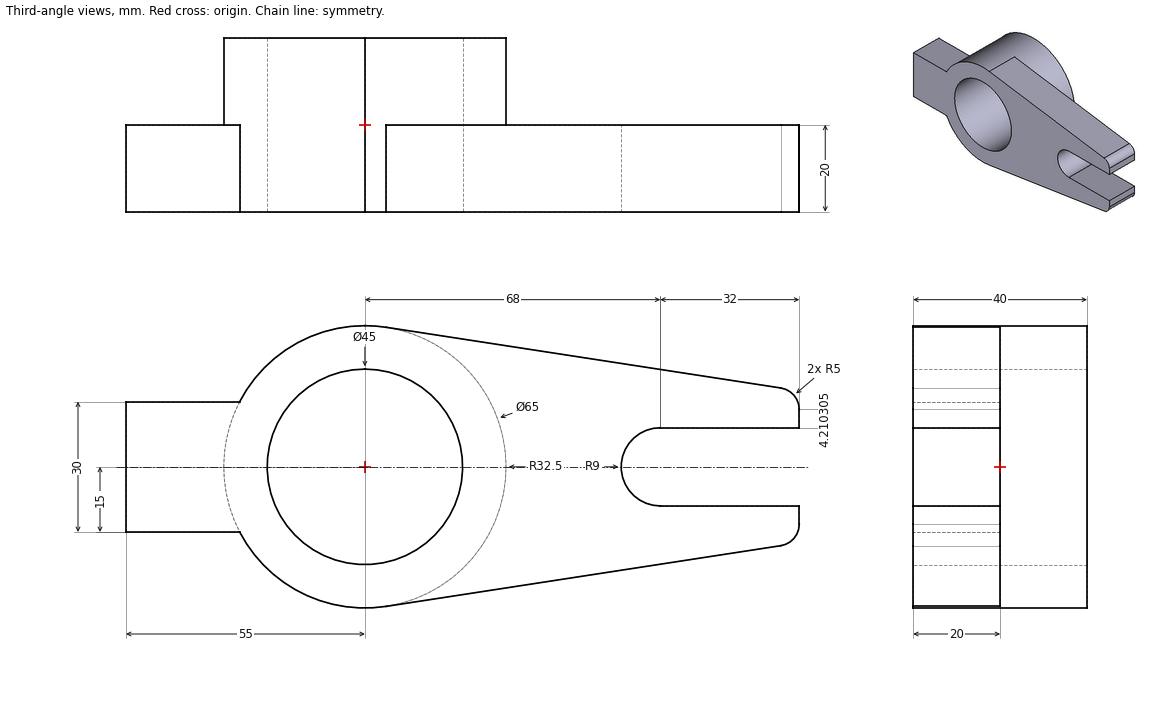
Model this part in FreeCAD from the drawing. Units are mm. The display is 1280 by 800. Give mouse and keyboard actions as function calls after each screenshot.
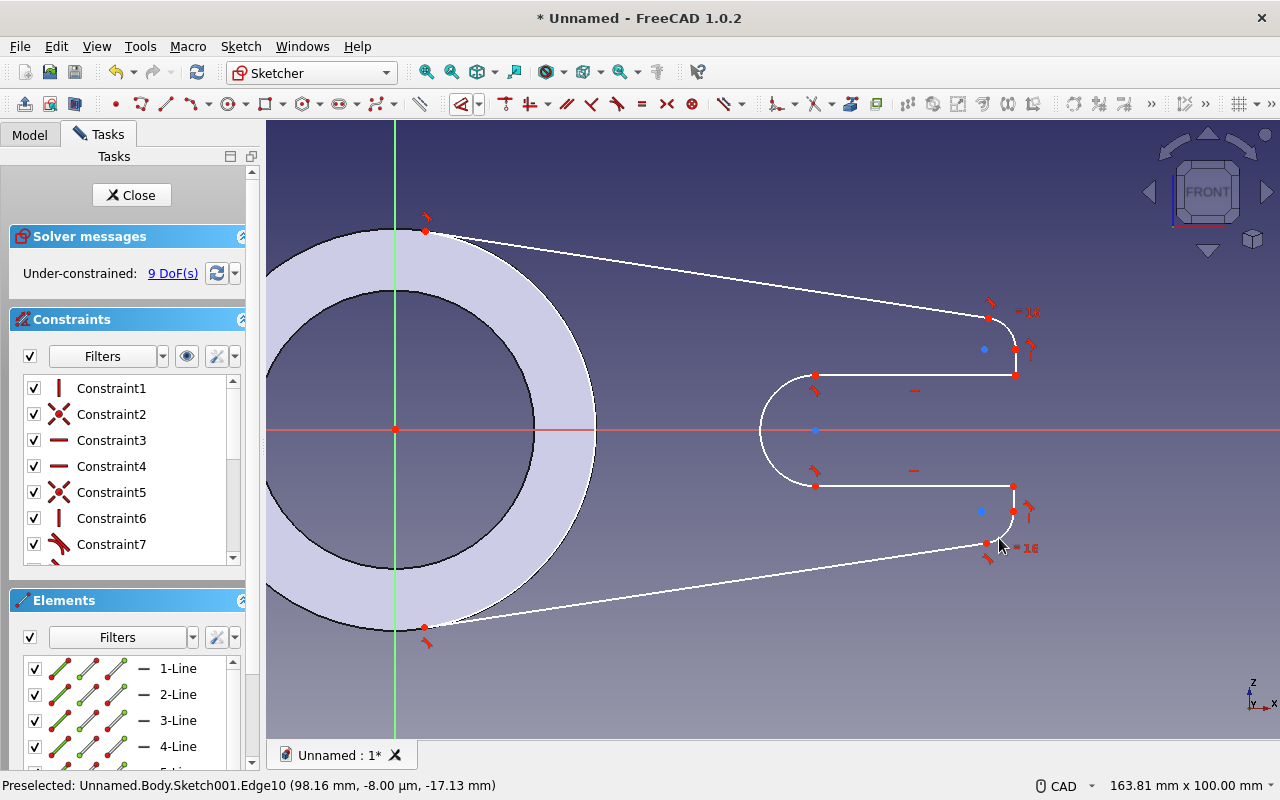
click(816, 431)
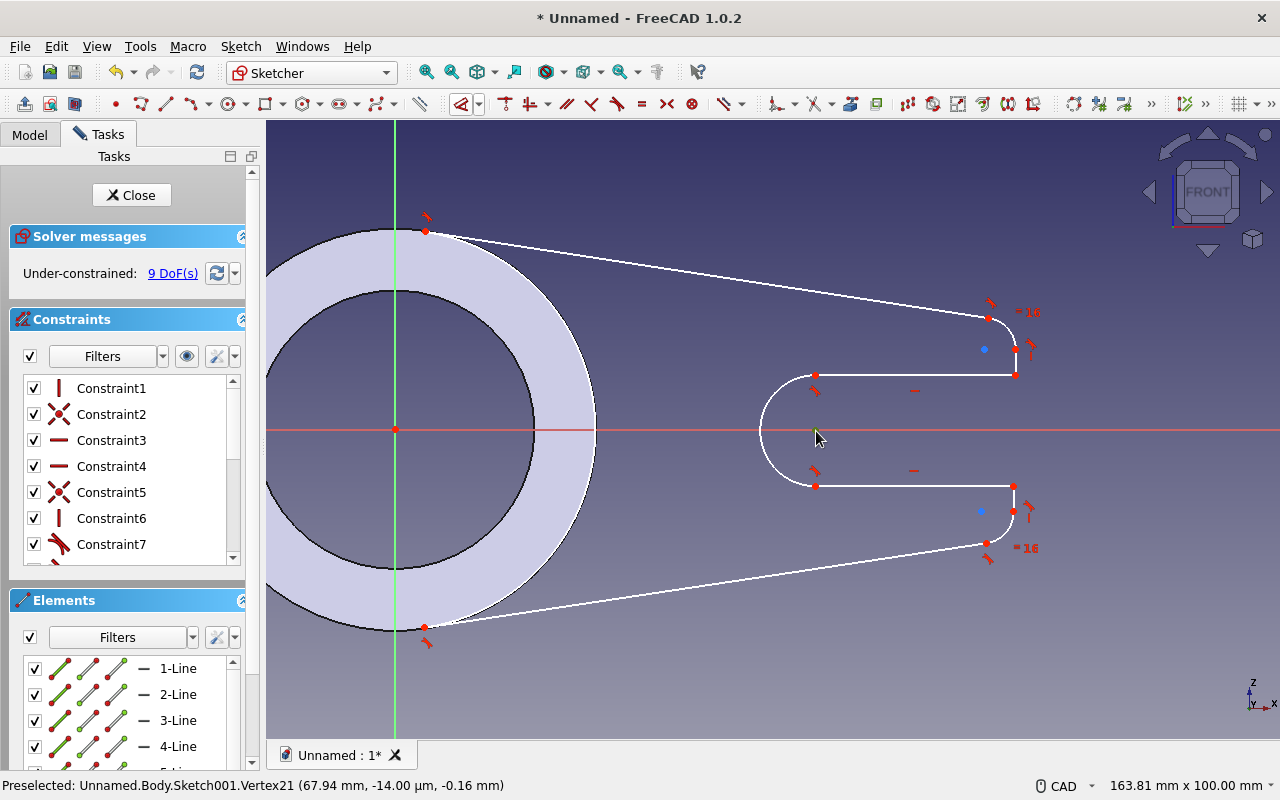
click(353, 430)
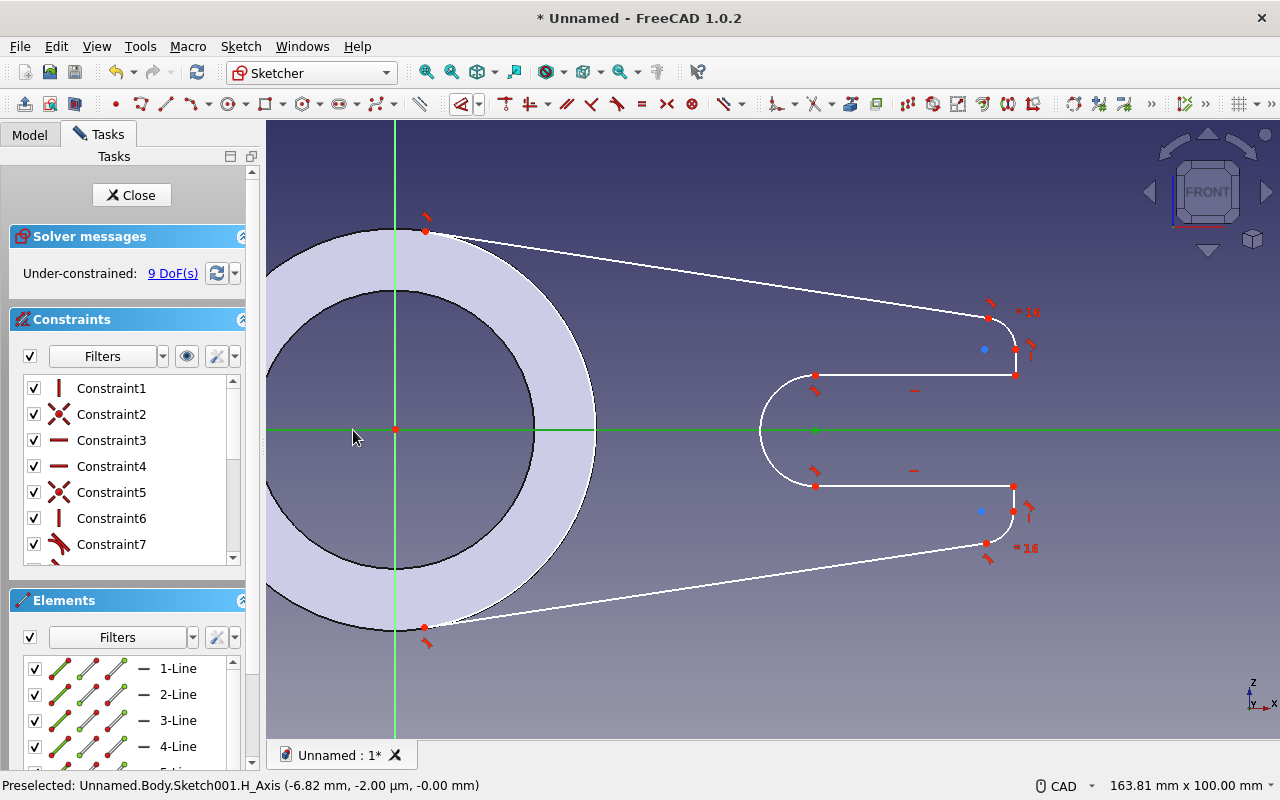
key(c)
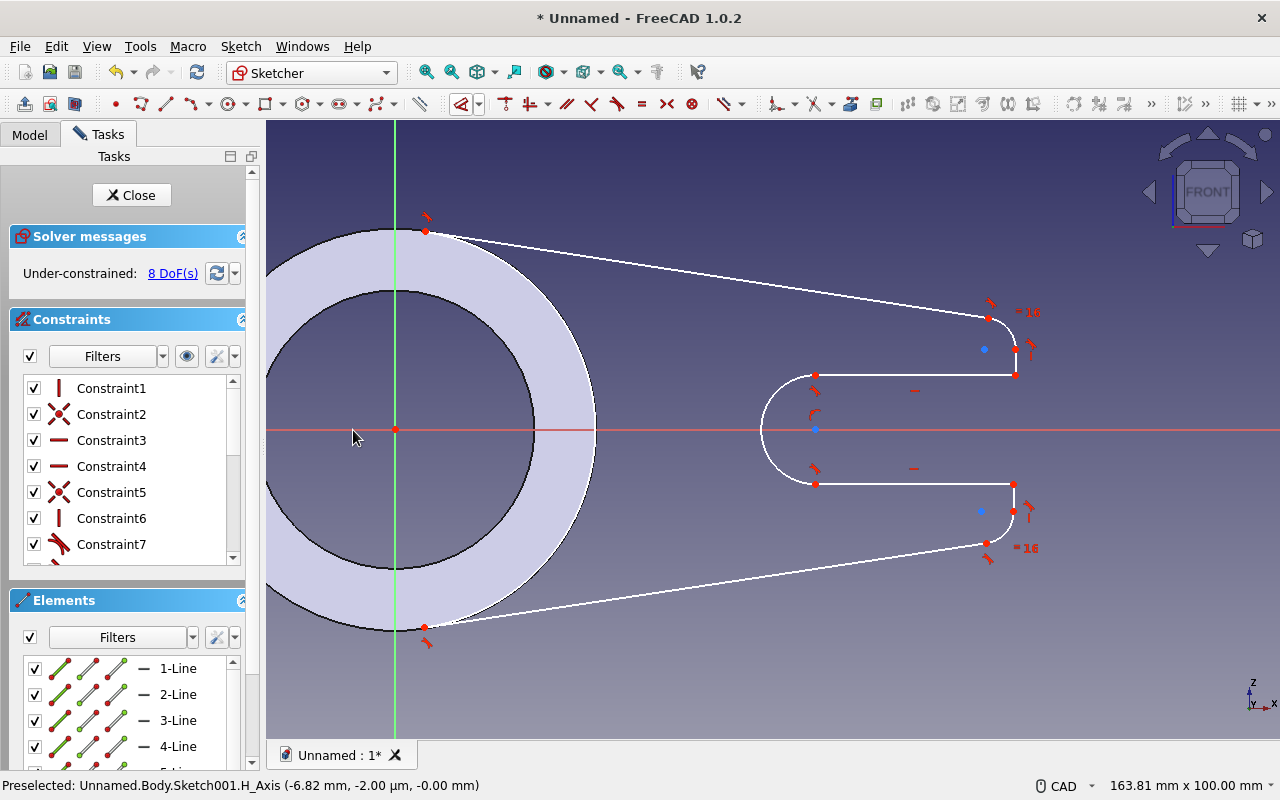
click(984, 349)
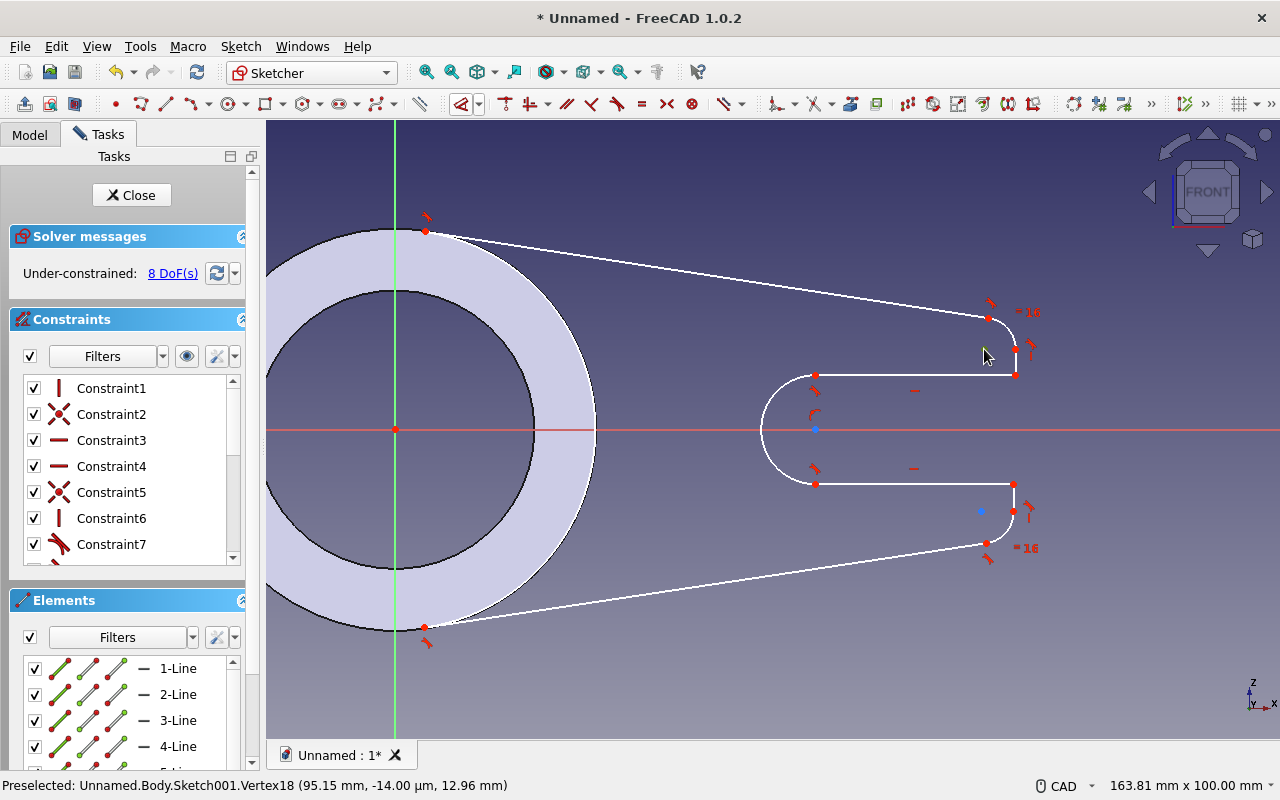
click(982, 512)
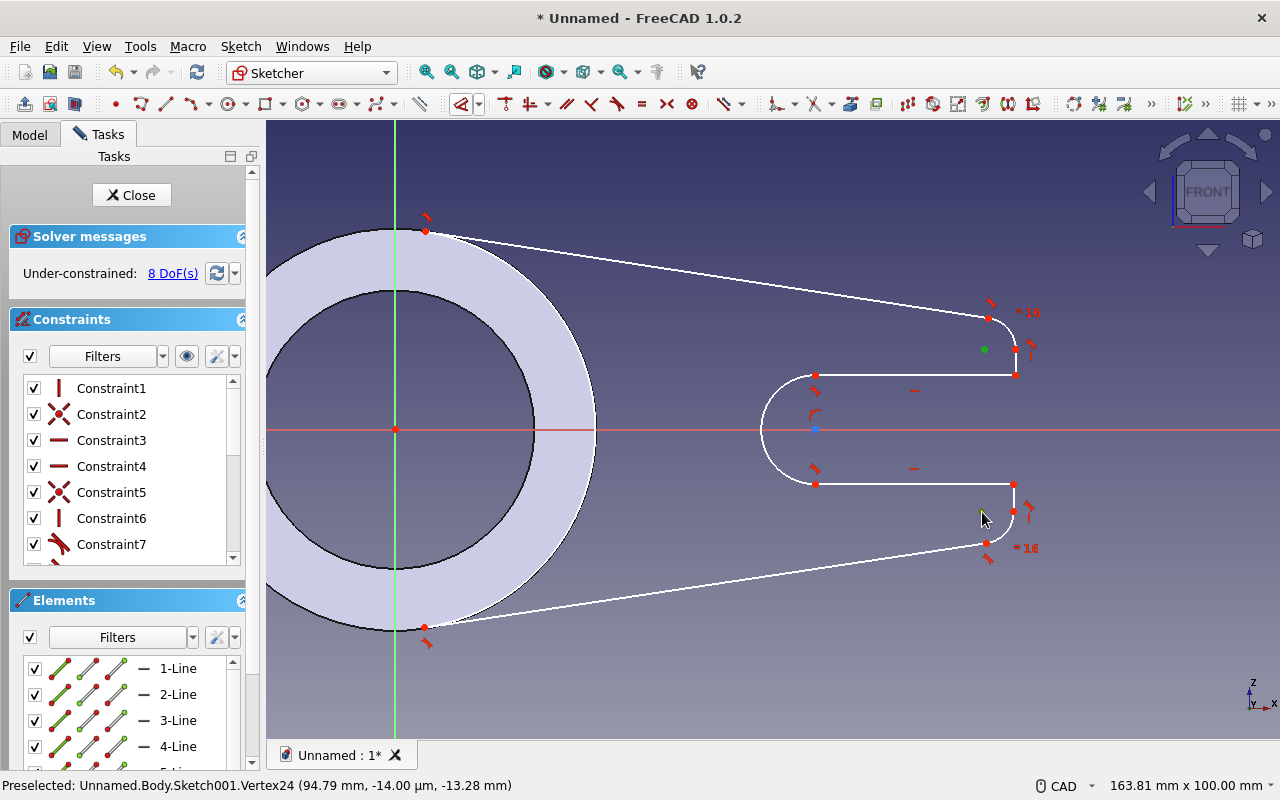
click(353, 430)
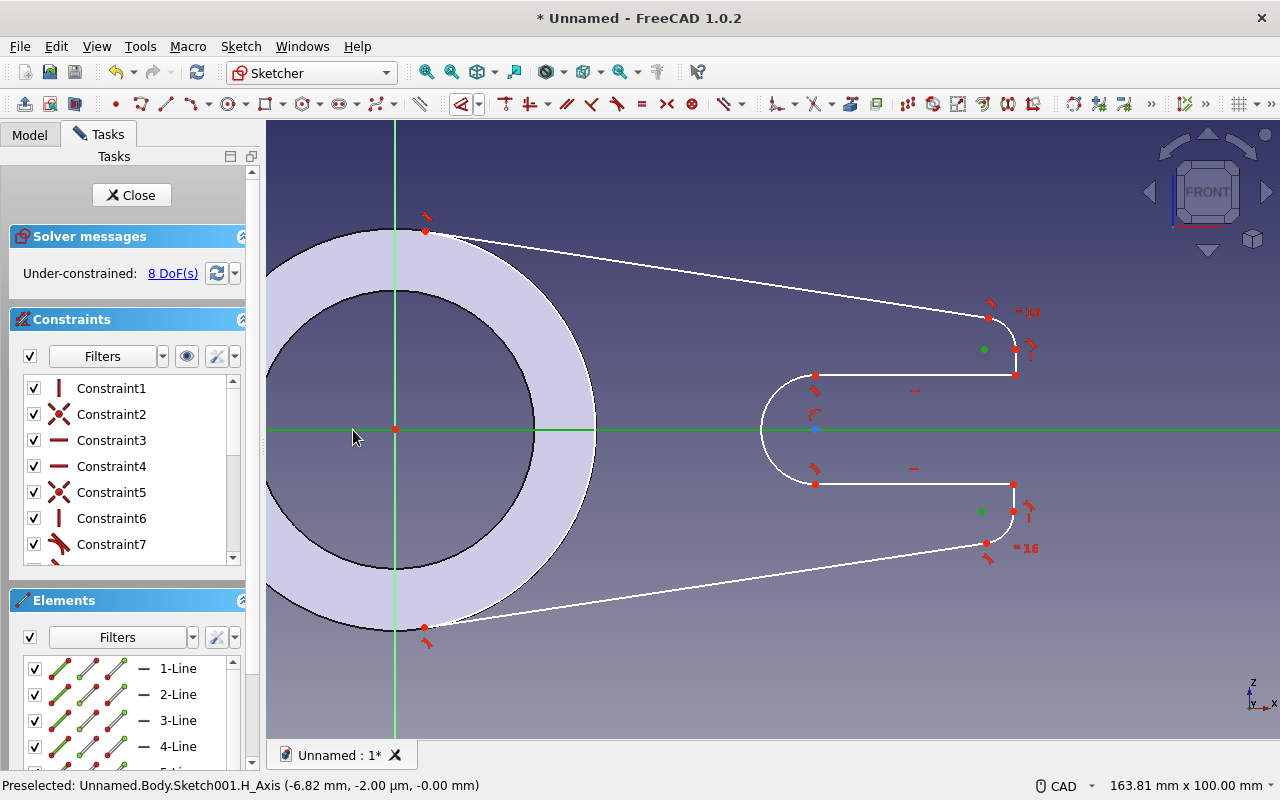
key(s)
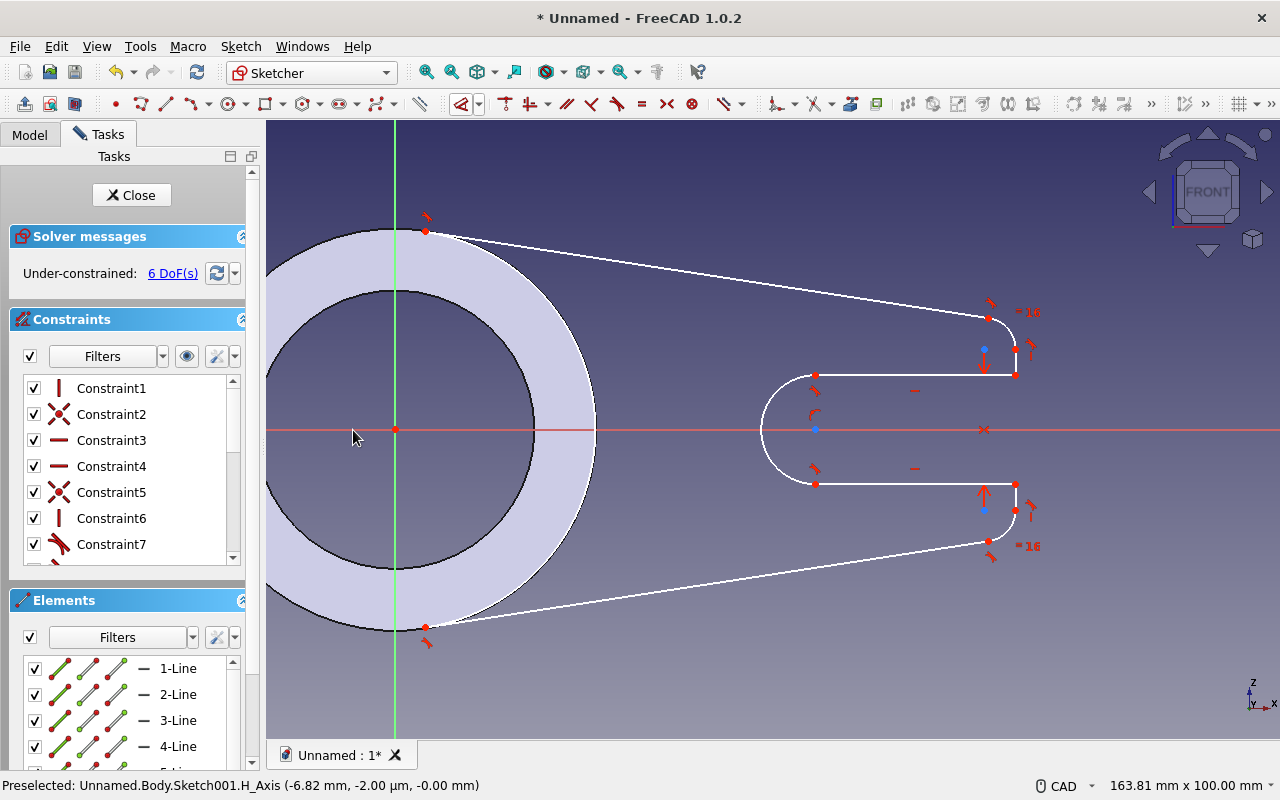
click(460, 104)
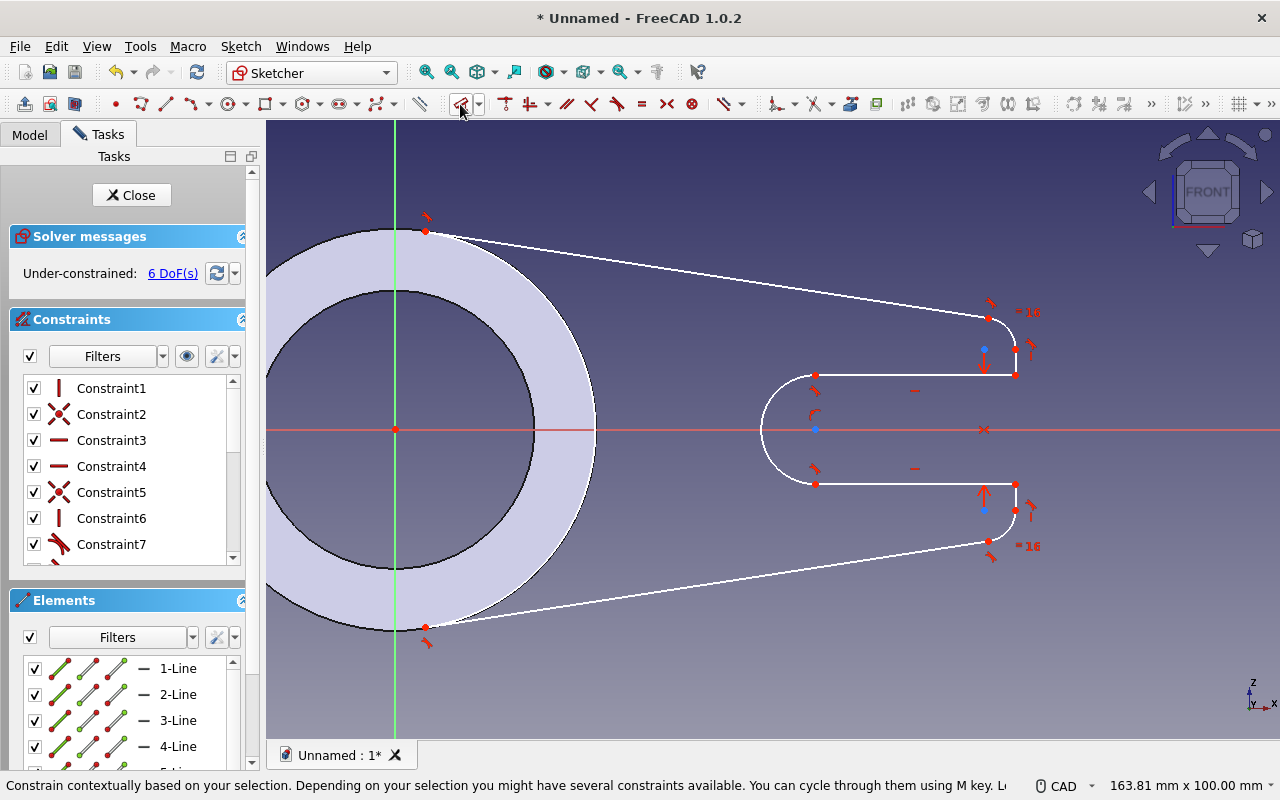
click(564, 537)
click(591, 554)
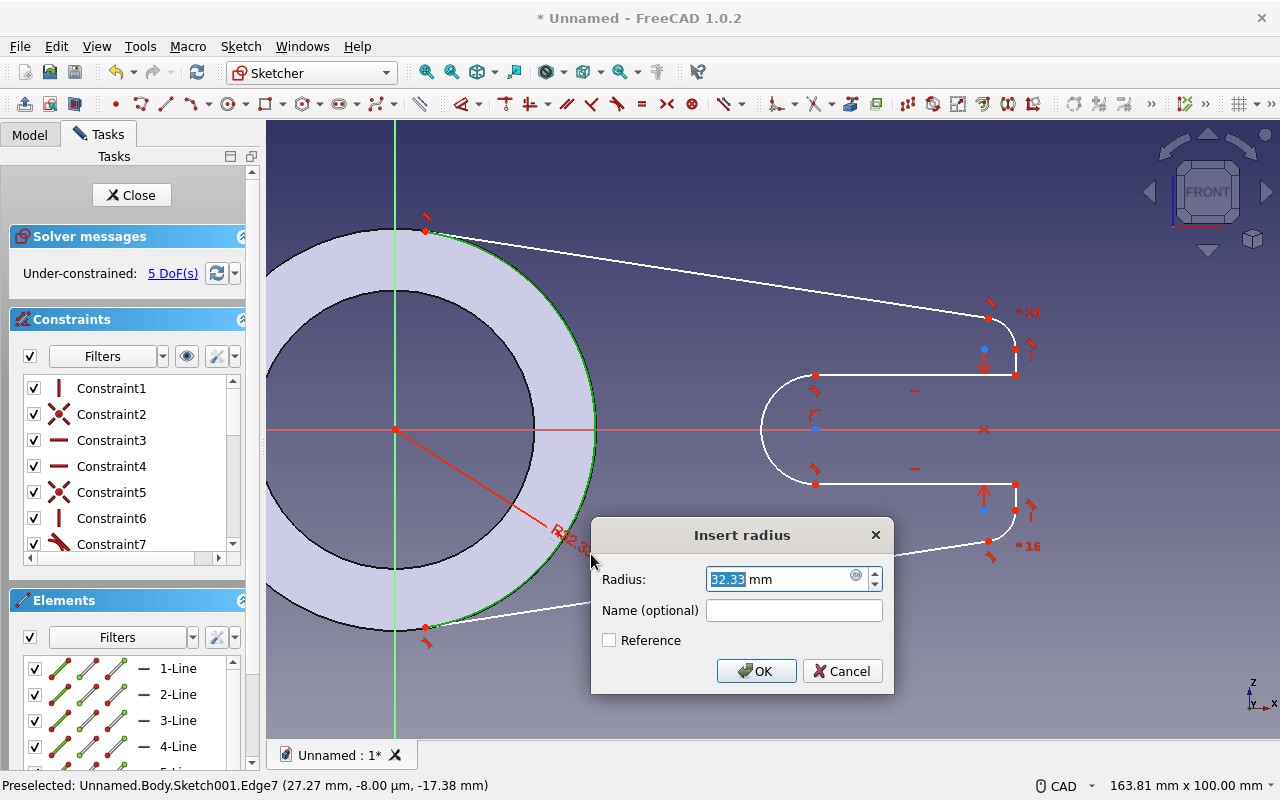
text(32.5)
key(Return)